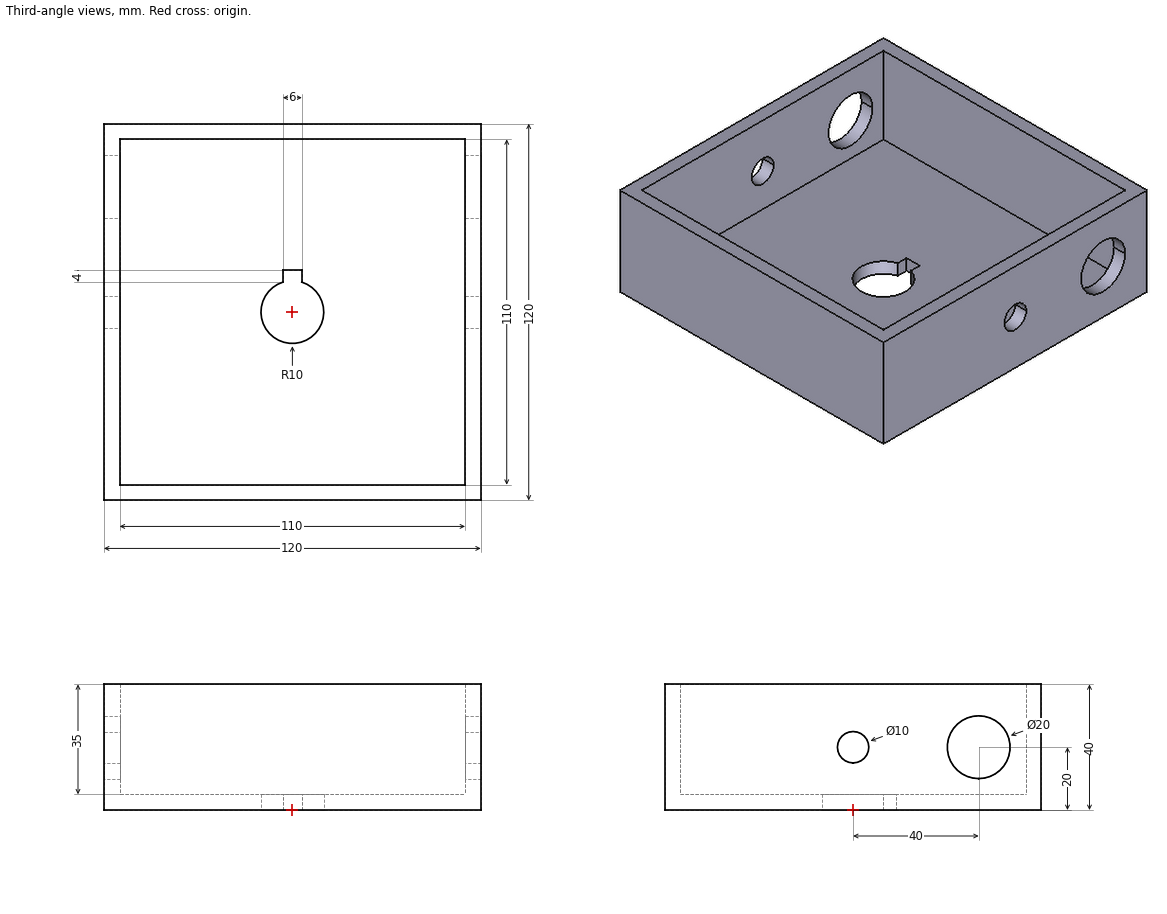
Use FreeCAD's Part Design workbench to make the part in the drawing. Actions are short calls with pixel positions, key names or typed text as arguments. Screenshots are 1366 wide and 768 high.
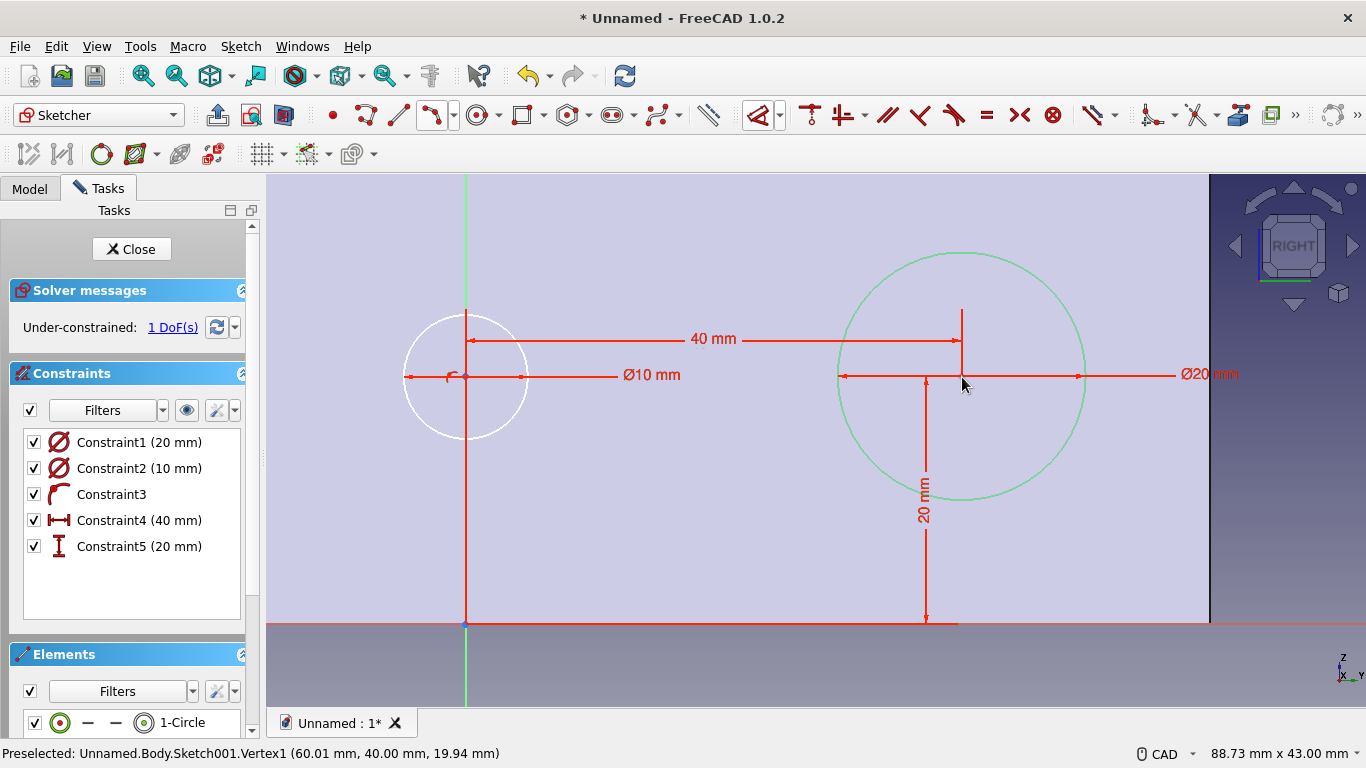
click(466, 377)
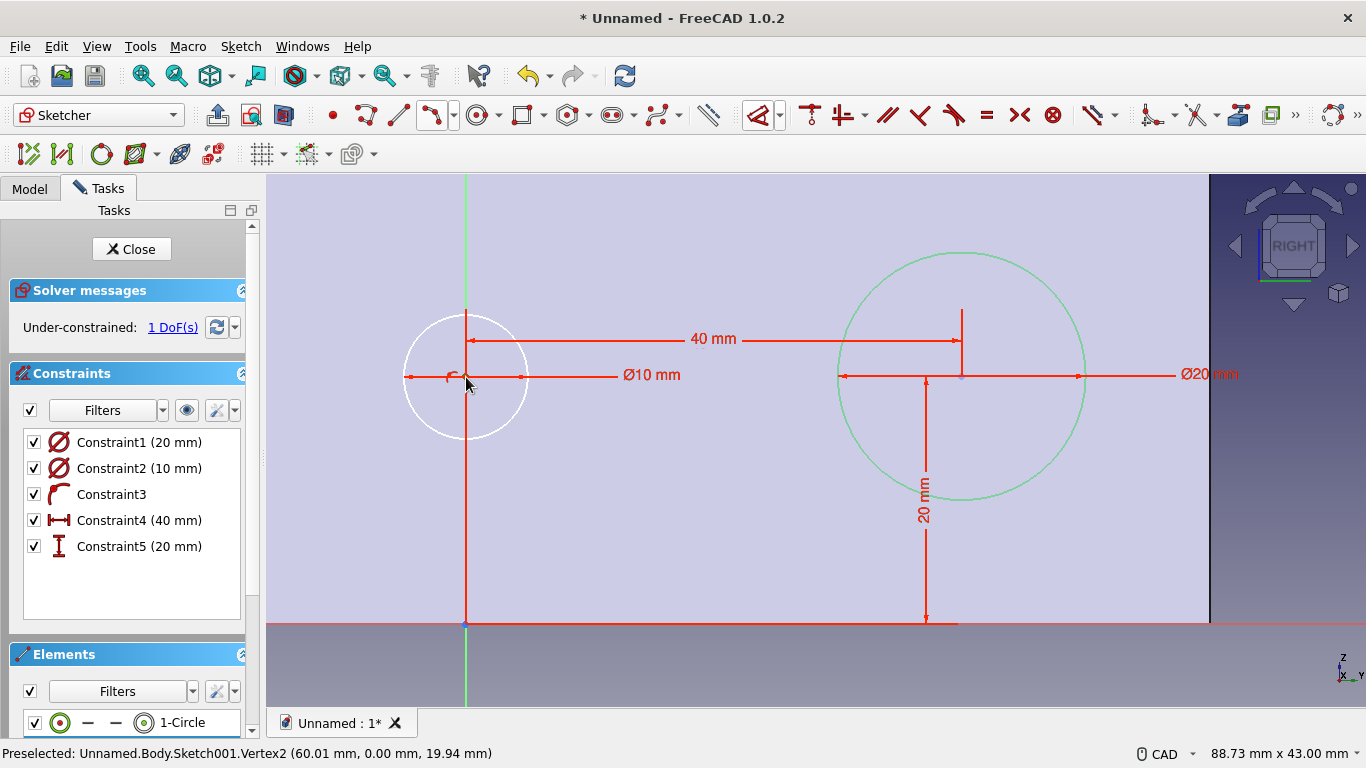
key(i)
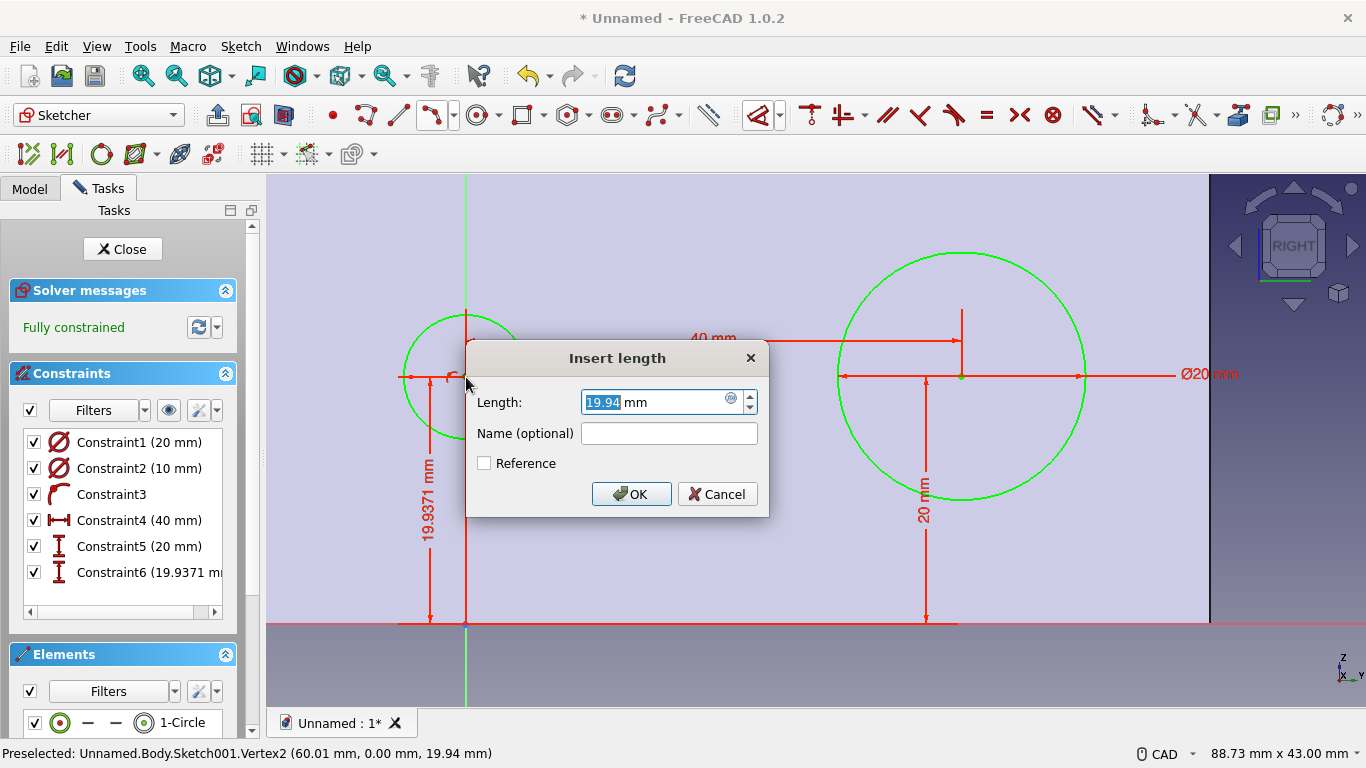
text(20)
key(Return)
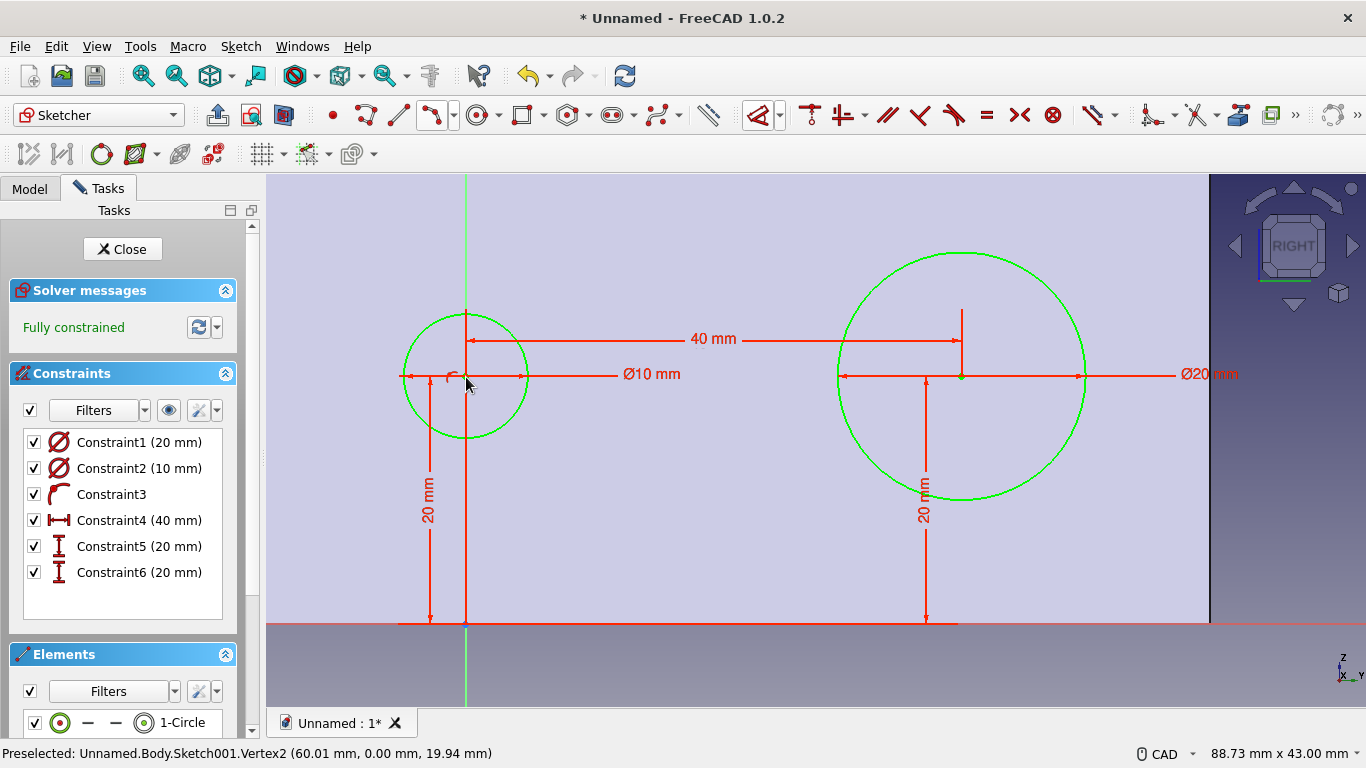
click(123, 249)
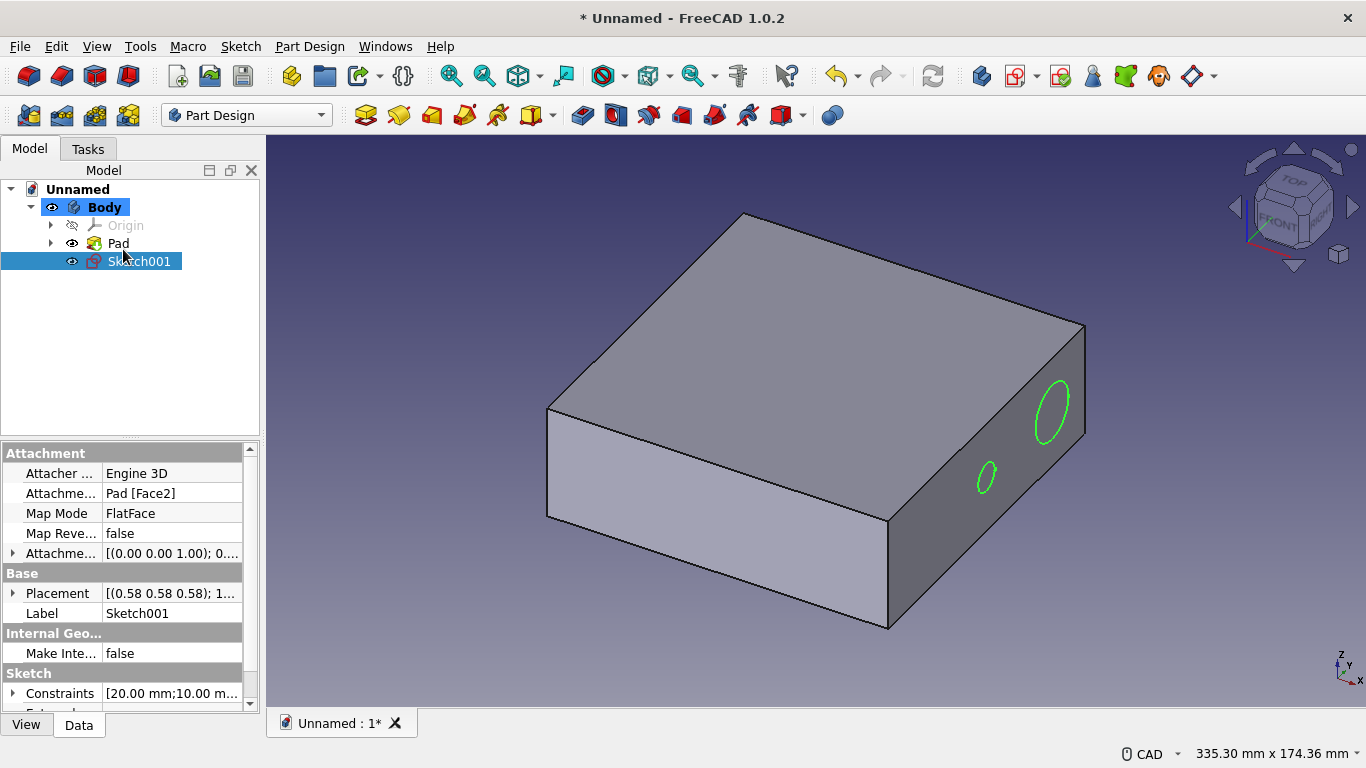
click(583, 116)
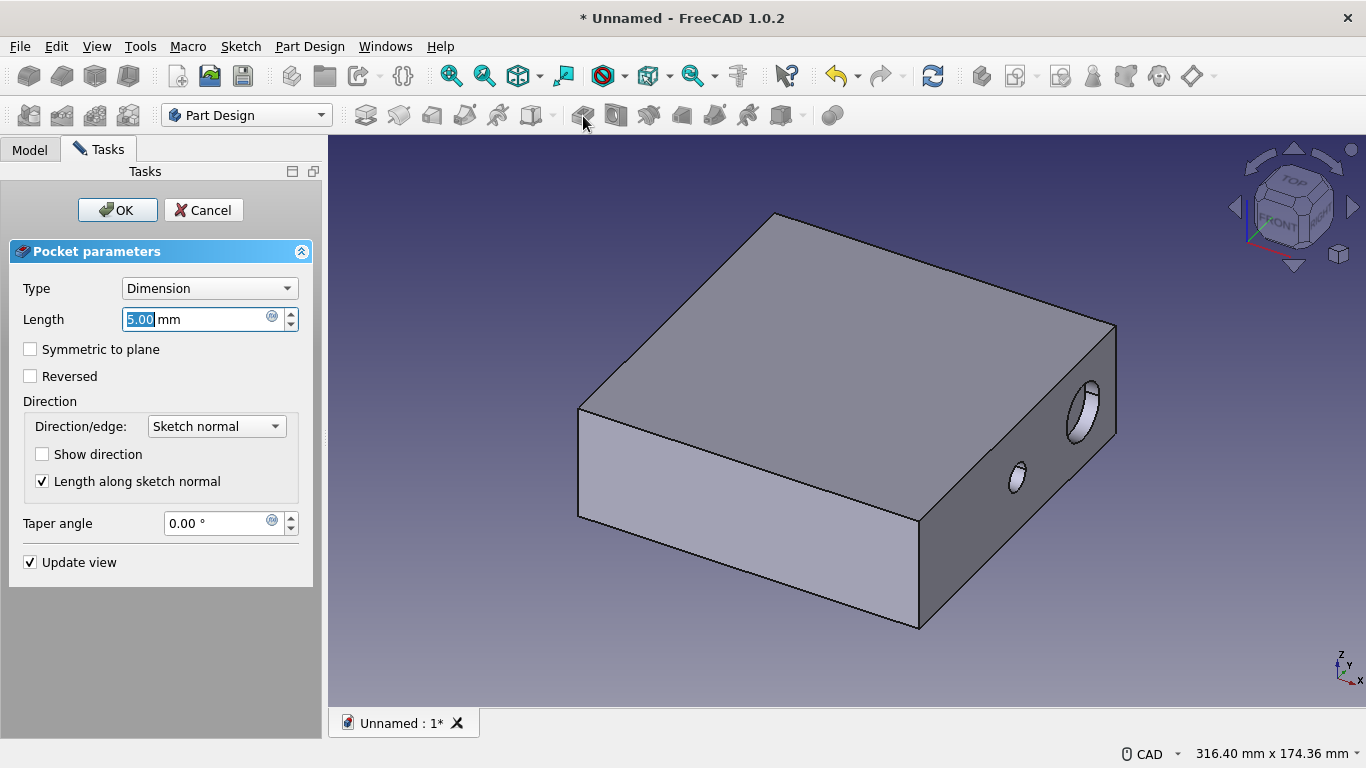
click(210, 288)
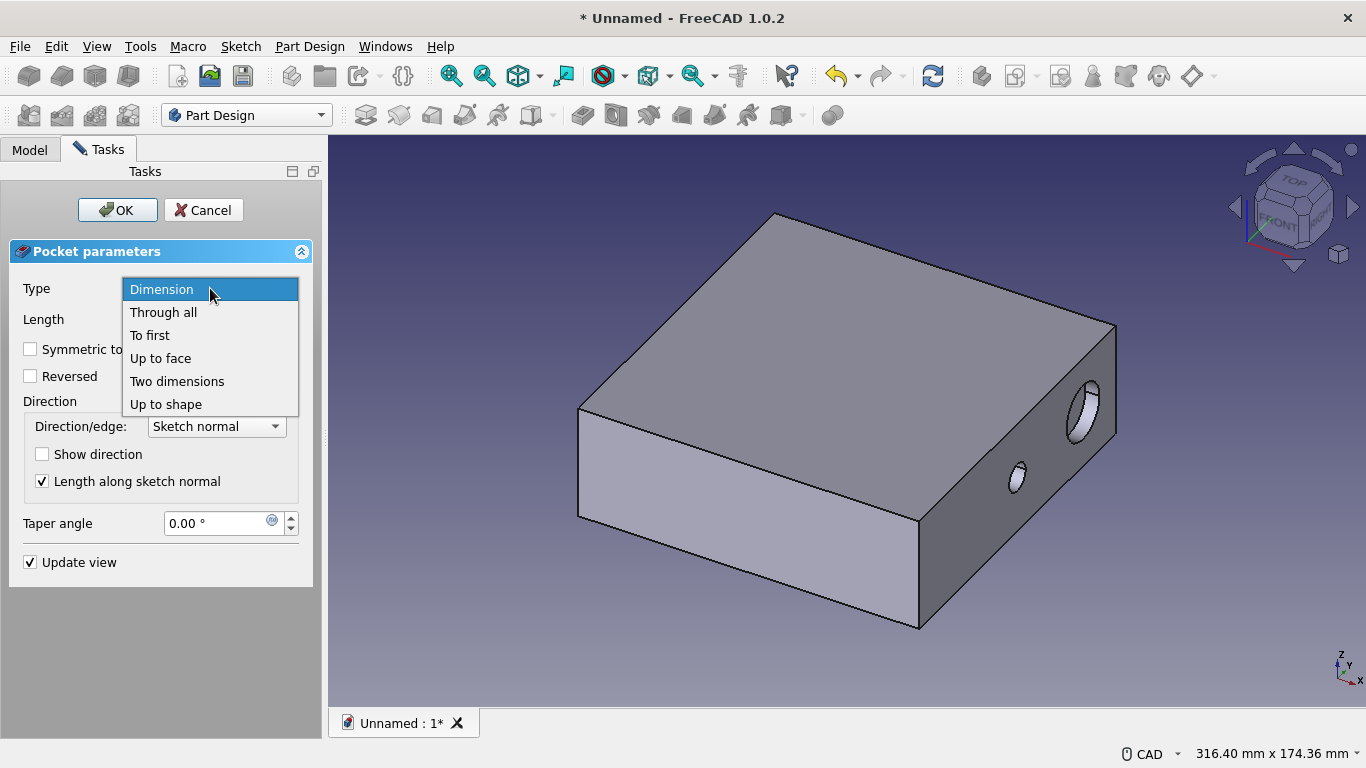
click(208, 312)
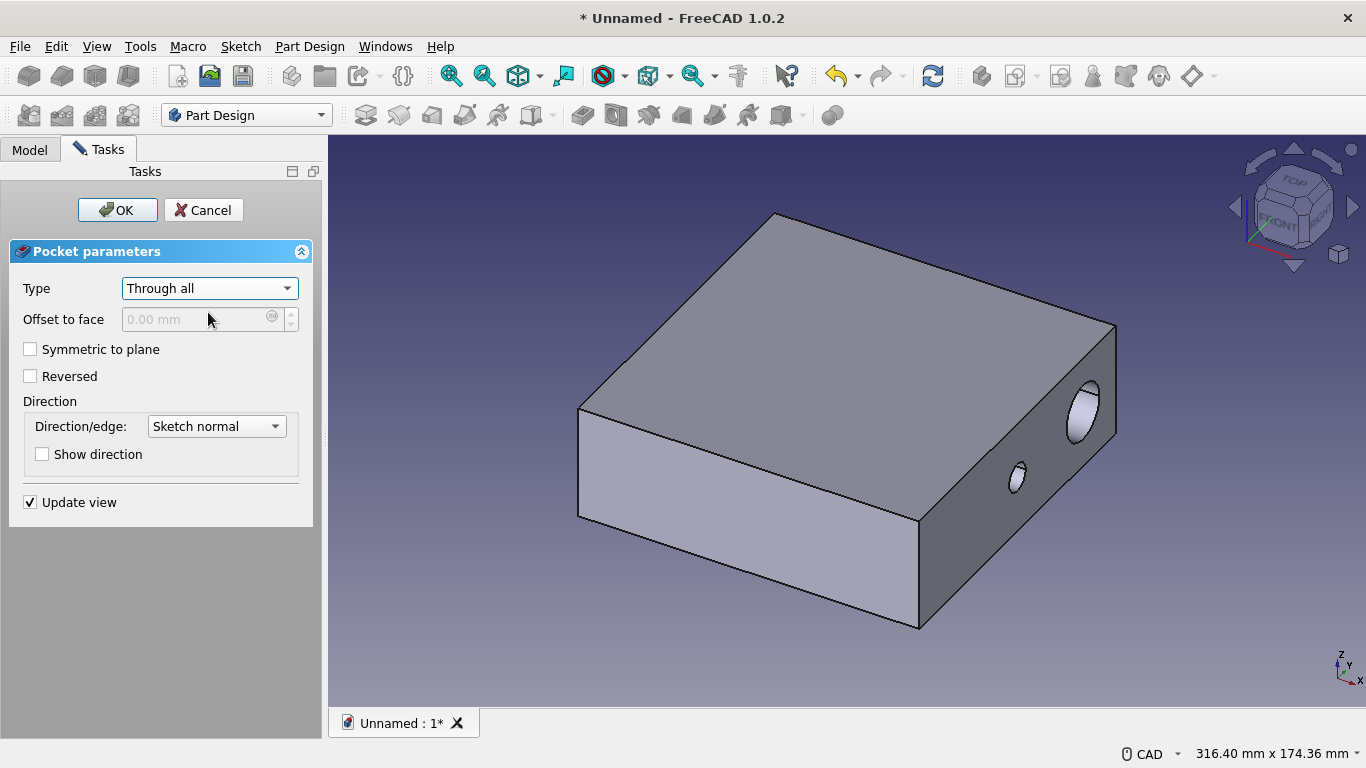
click(118, 210)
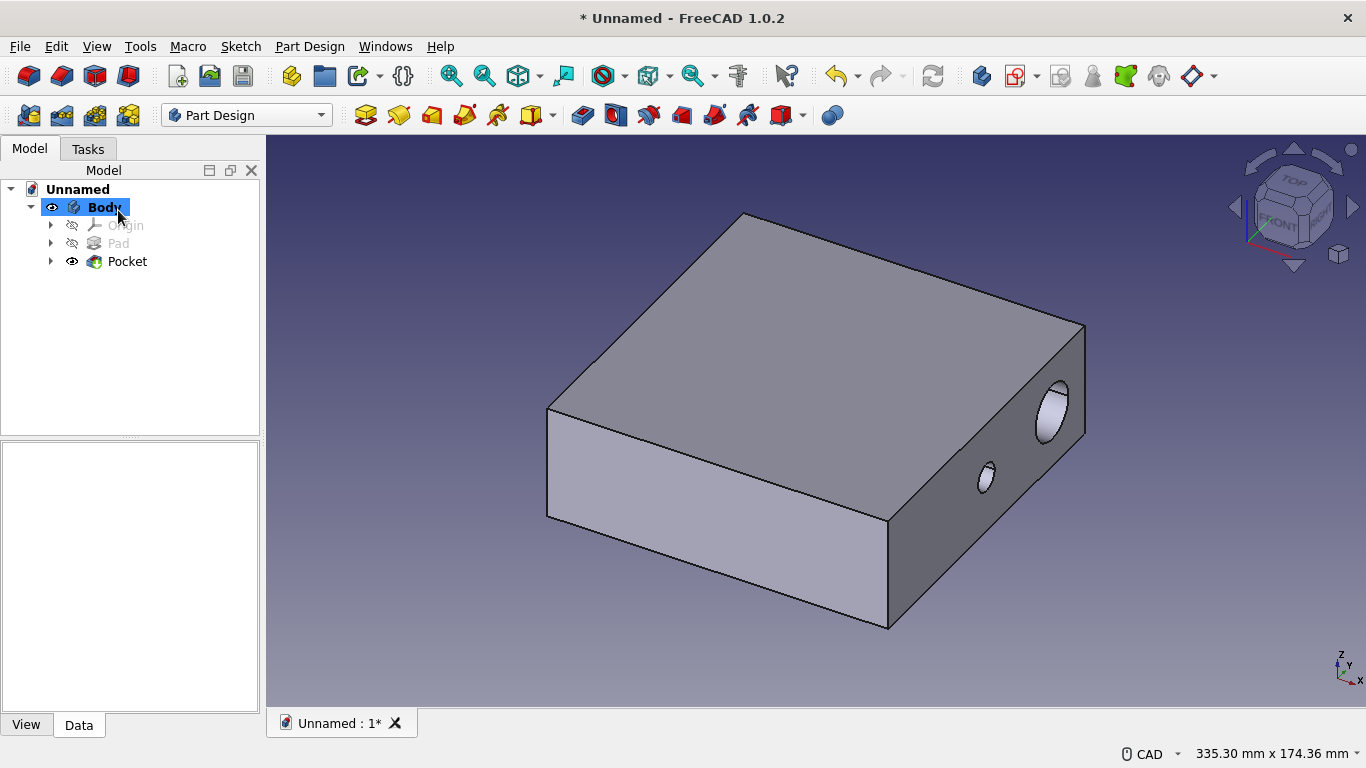
click(816, 366)